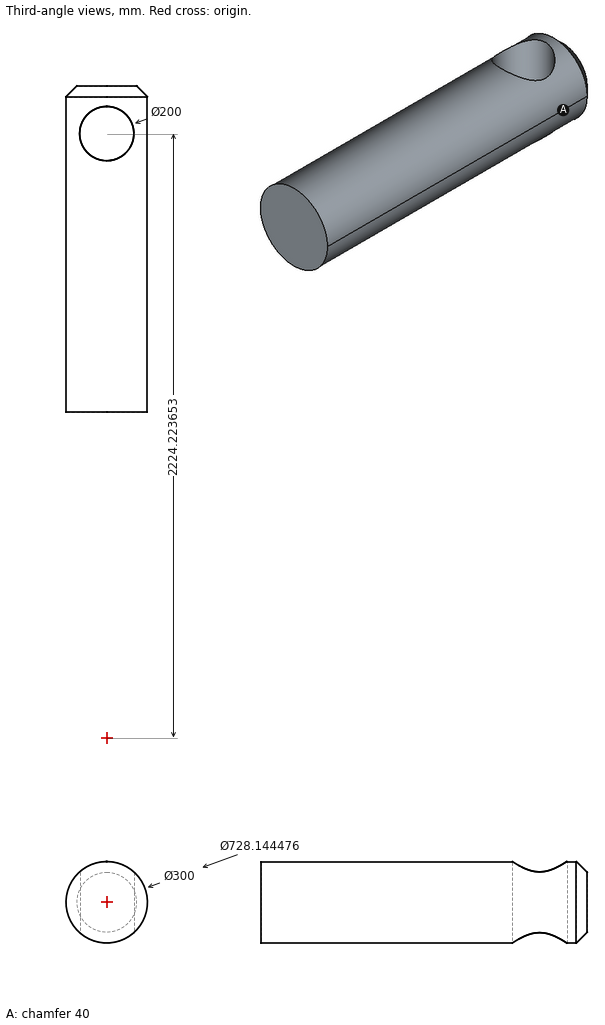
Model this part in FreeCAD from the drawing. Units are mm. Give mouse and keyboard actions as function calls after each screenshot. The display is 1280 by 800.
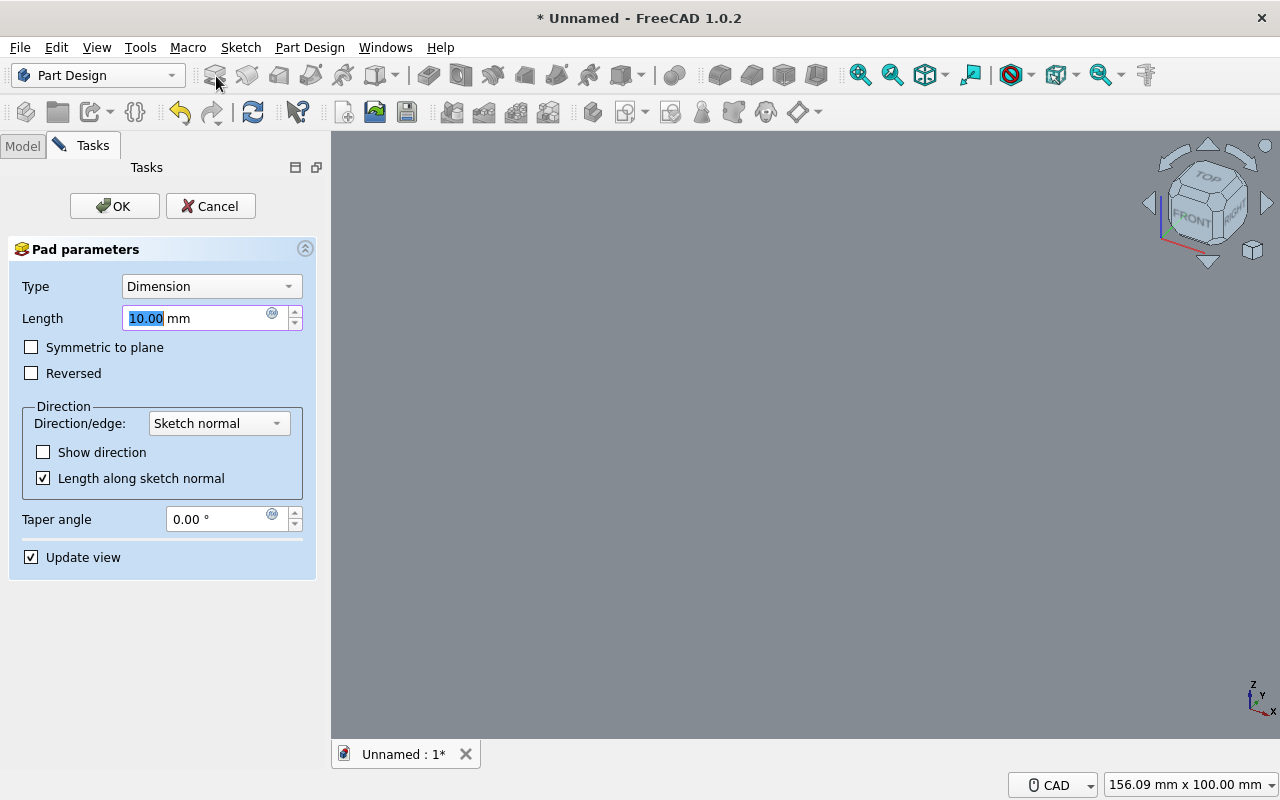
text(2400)
key(Tab)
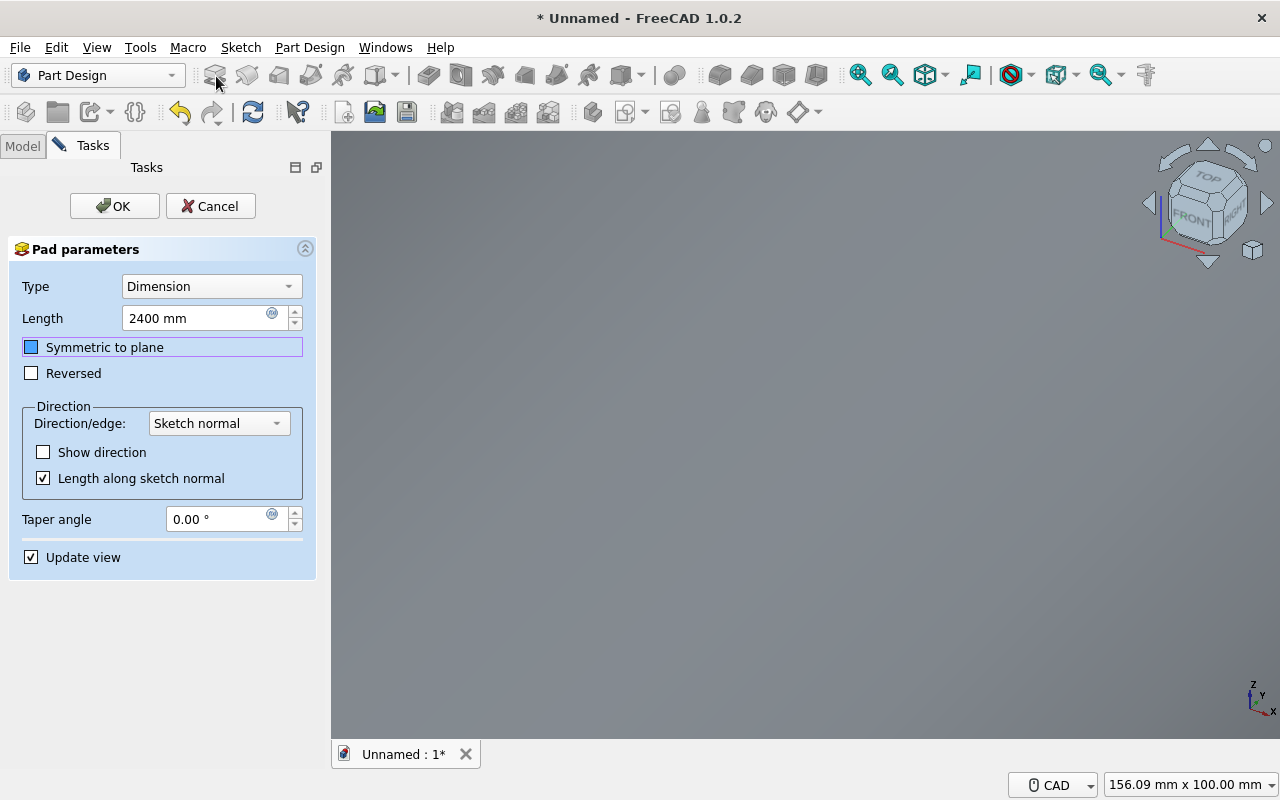
click(30, 373)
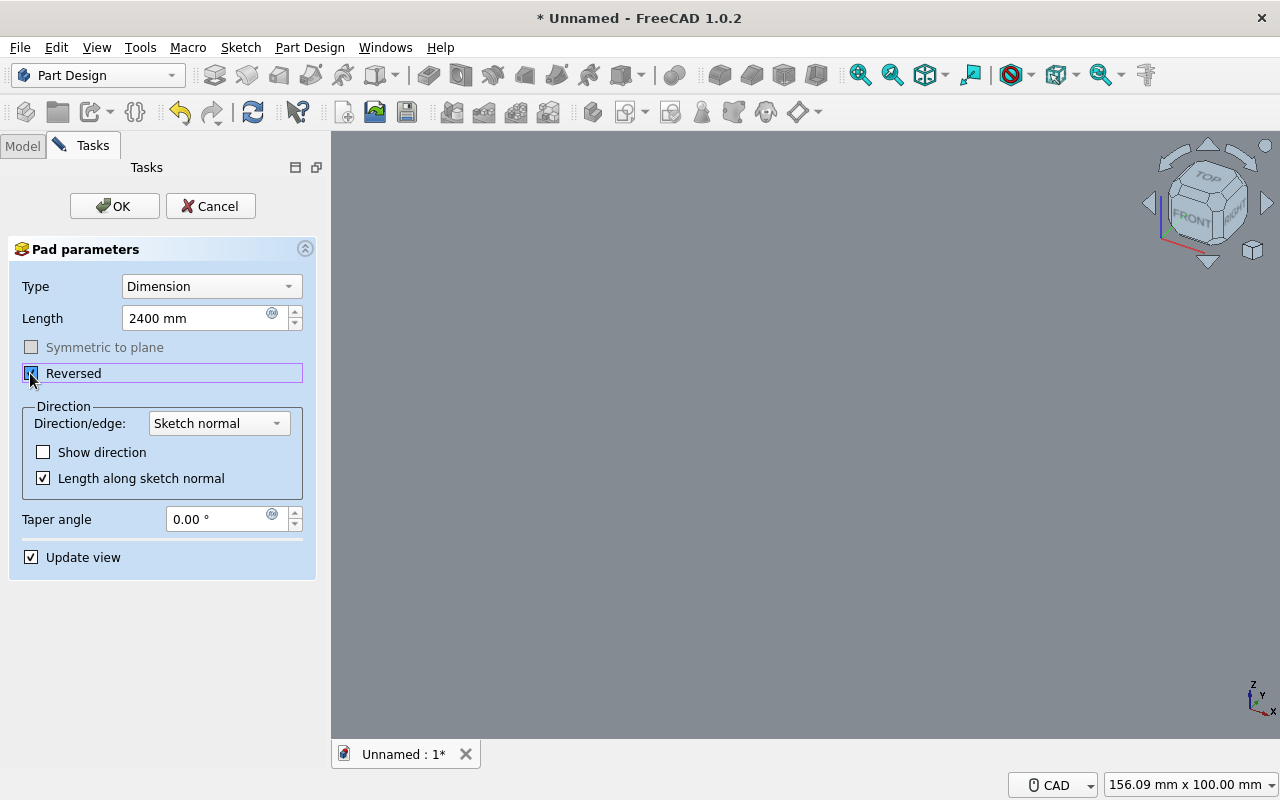
click(115, 206)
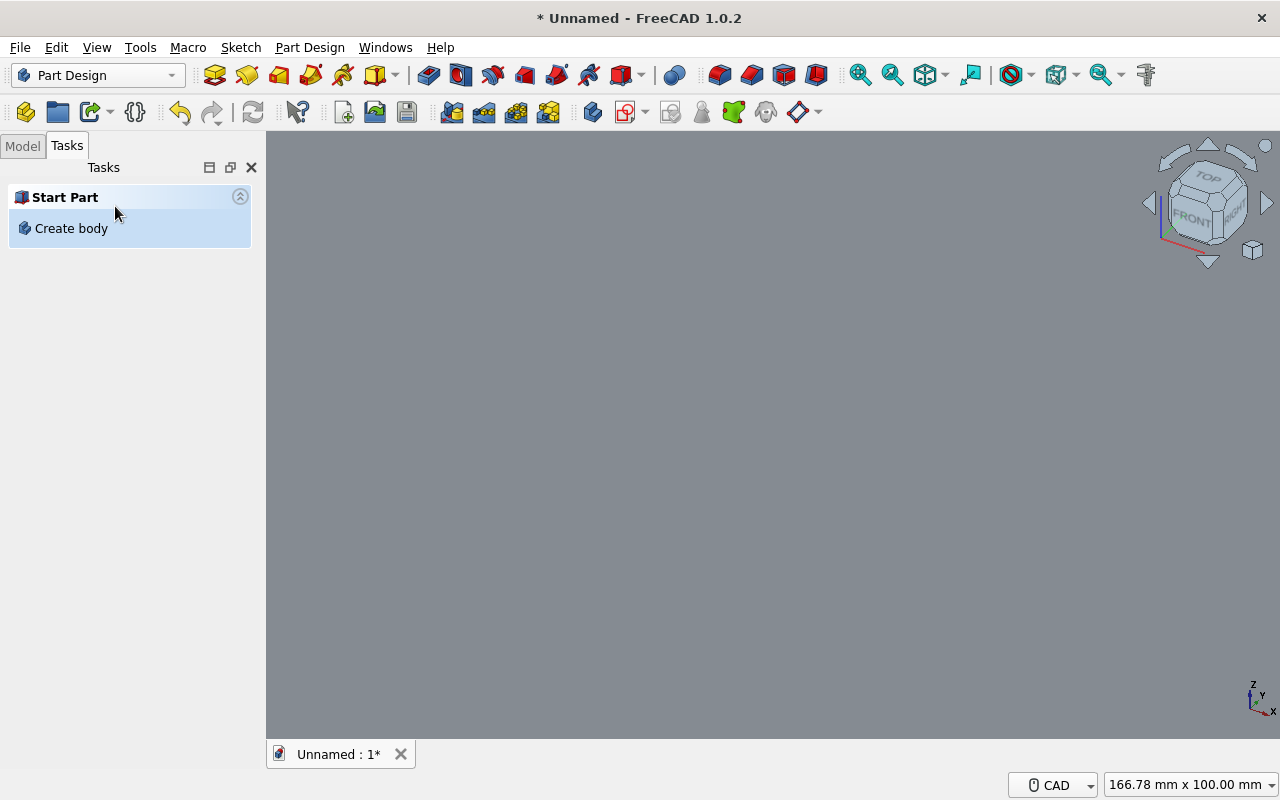
click(862, 76)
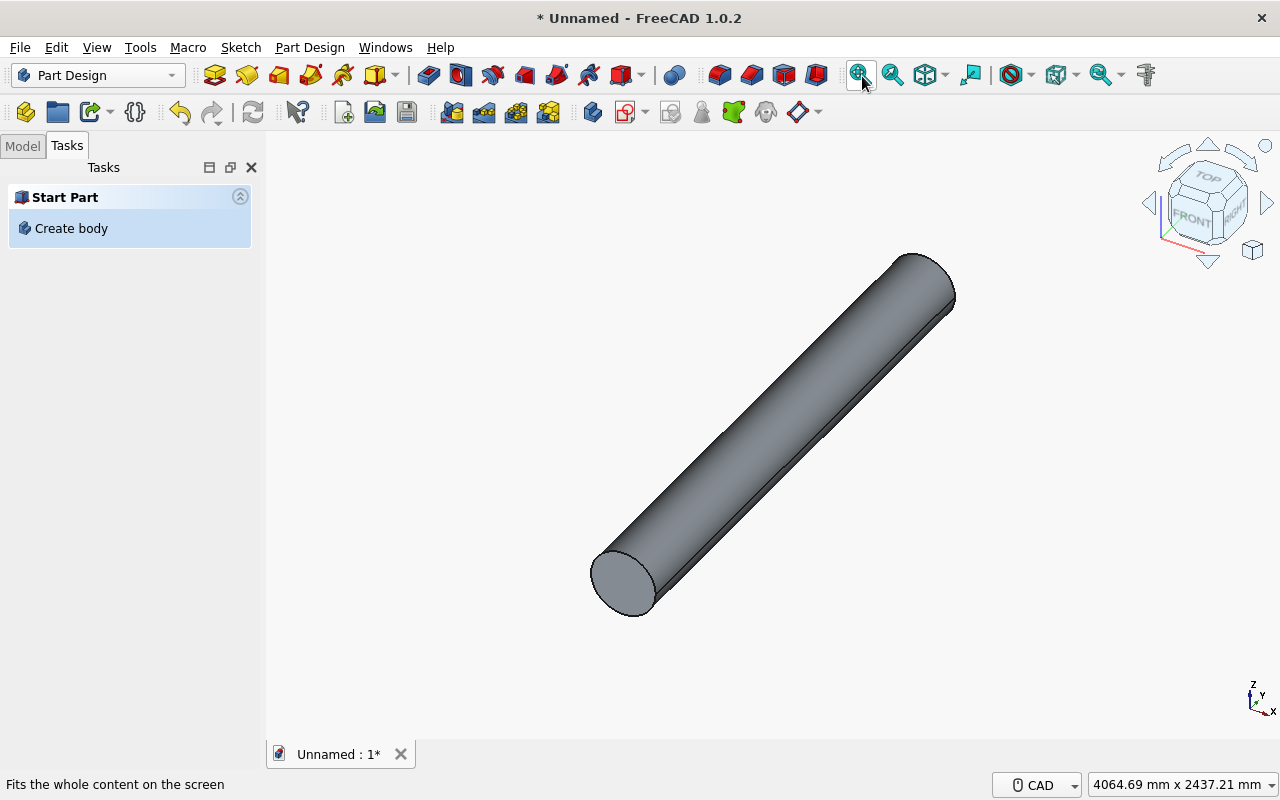
click(626, 112)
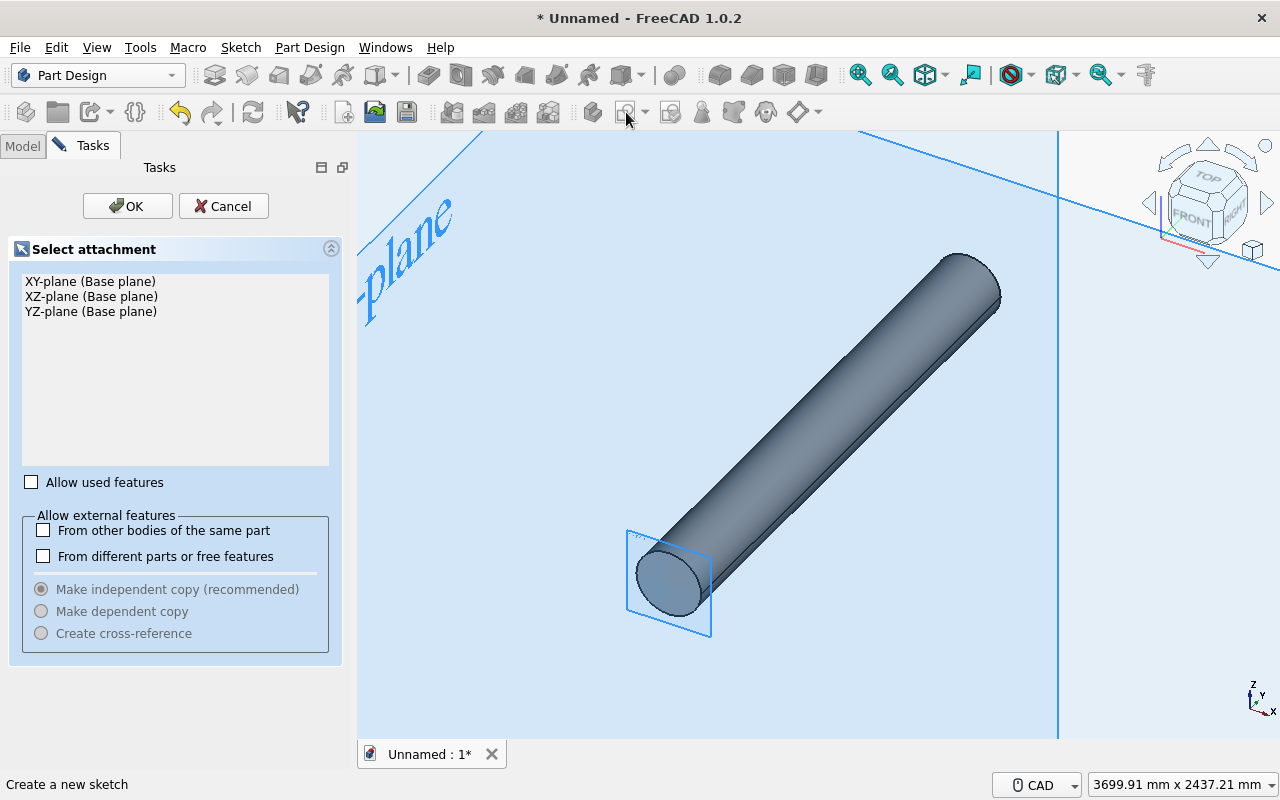
click(82, 282)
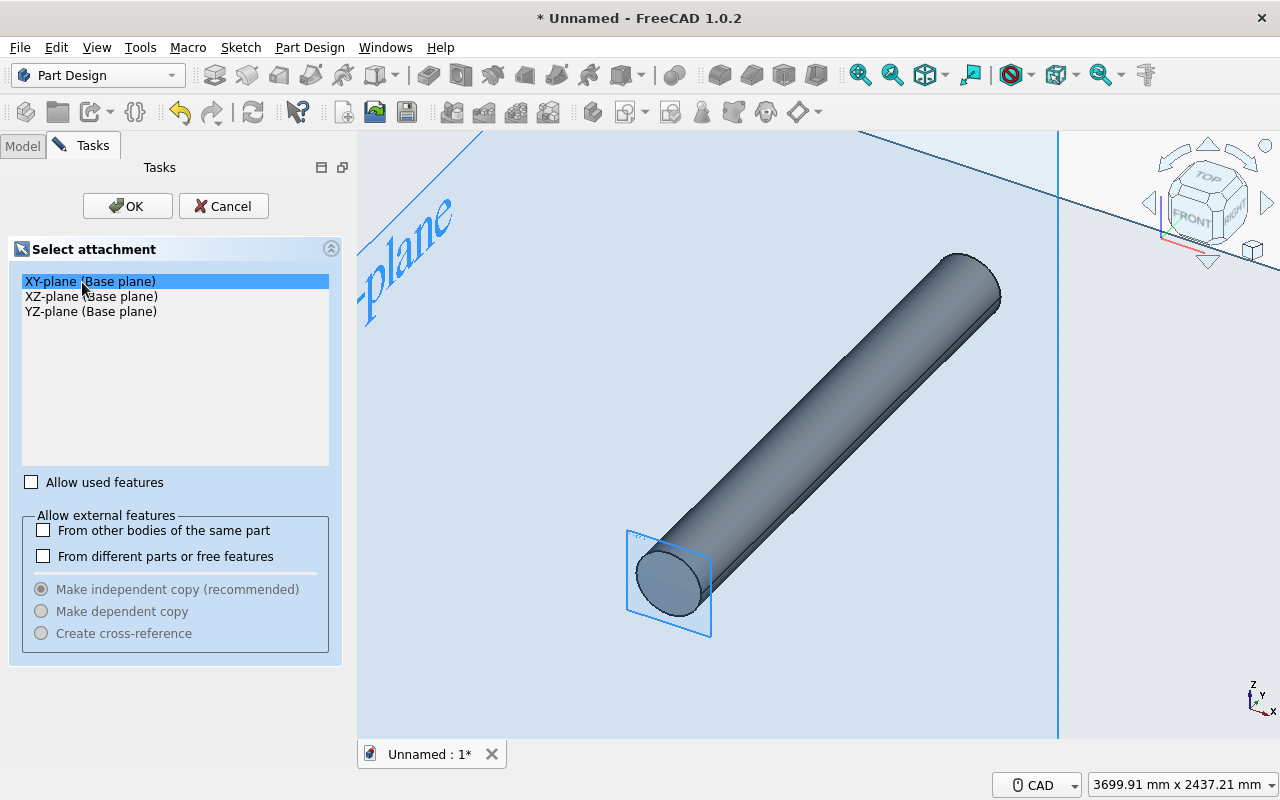
click(128, 206)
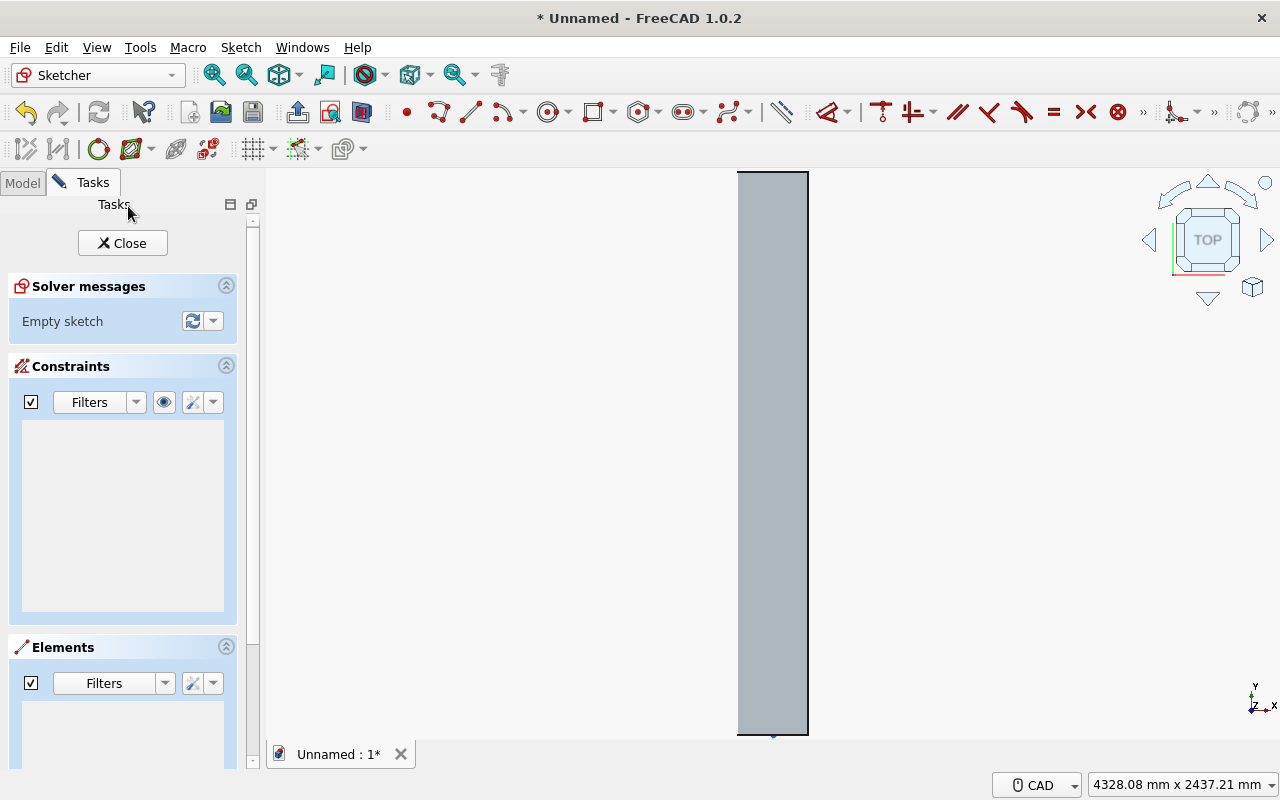
key(q)
key(s)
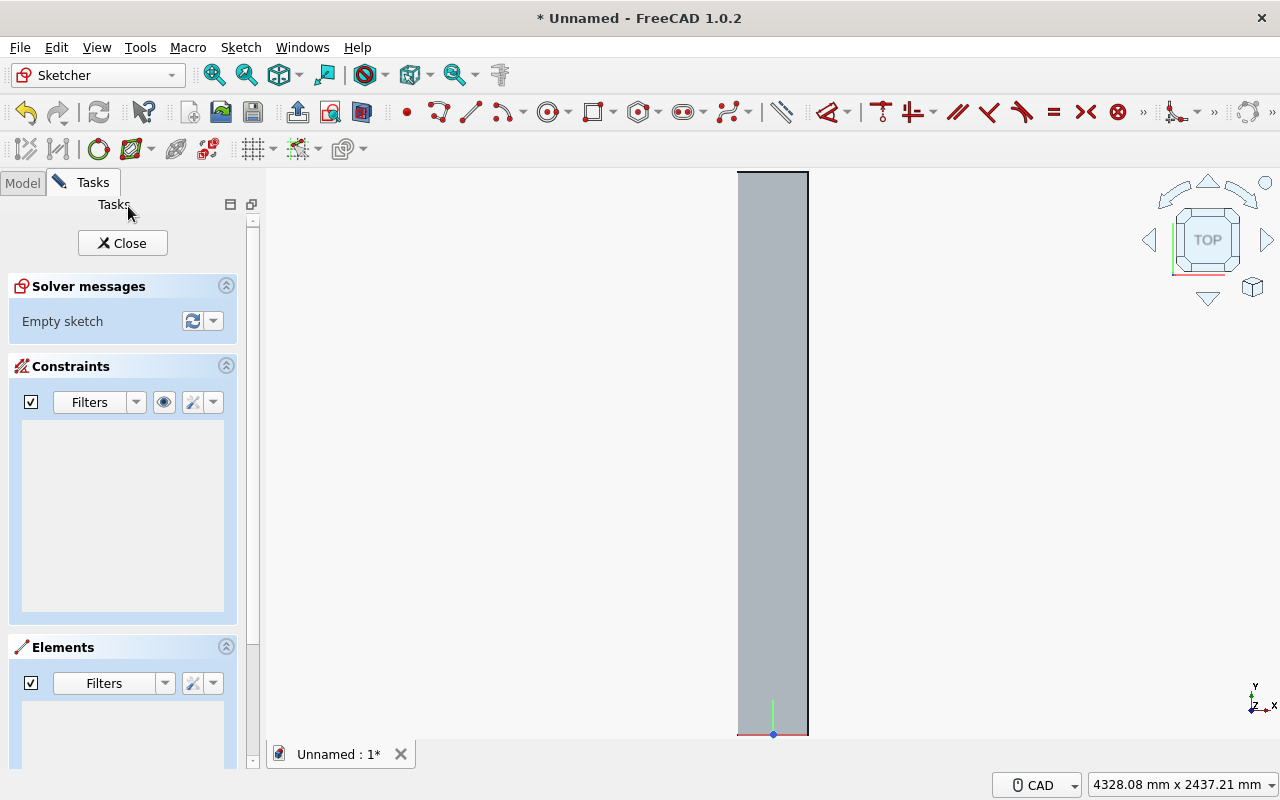
scroll(704, 454, down, 5)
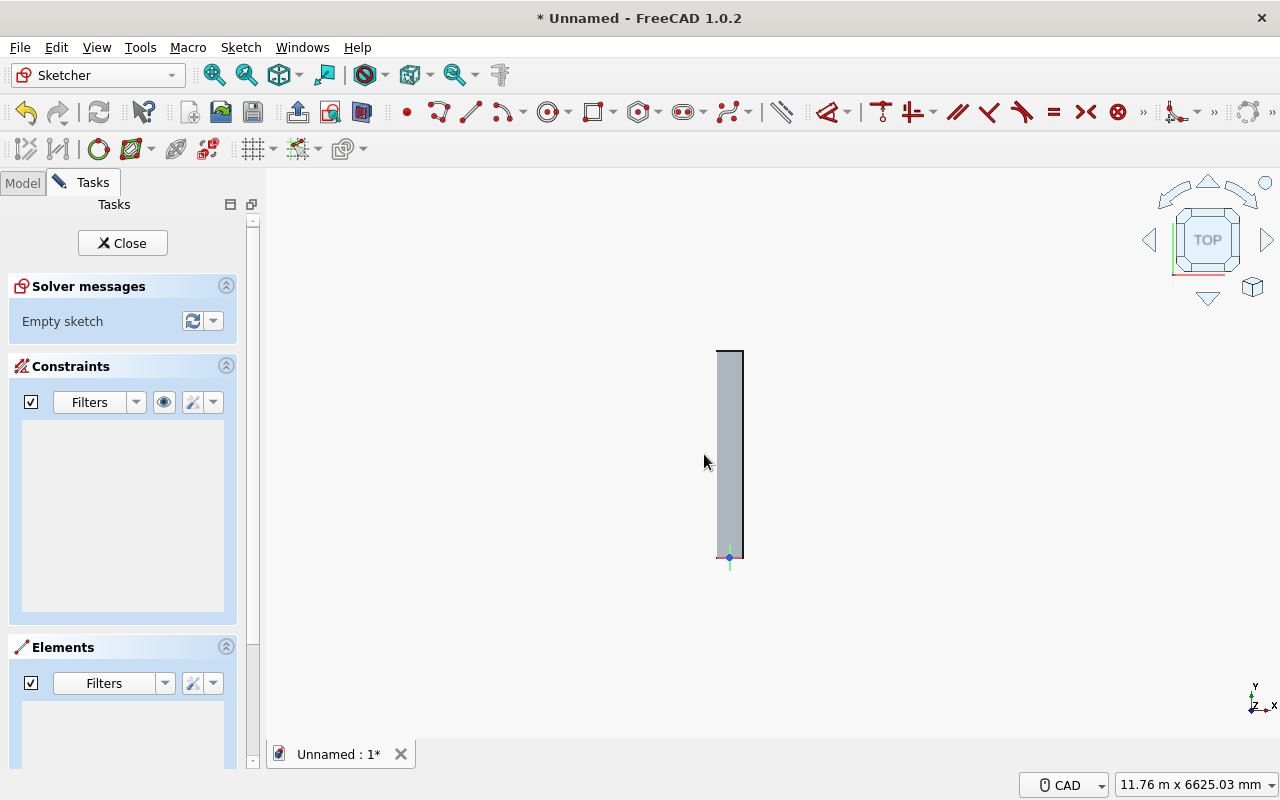
scroll(731, 361, up, 15)